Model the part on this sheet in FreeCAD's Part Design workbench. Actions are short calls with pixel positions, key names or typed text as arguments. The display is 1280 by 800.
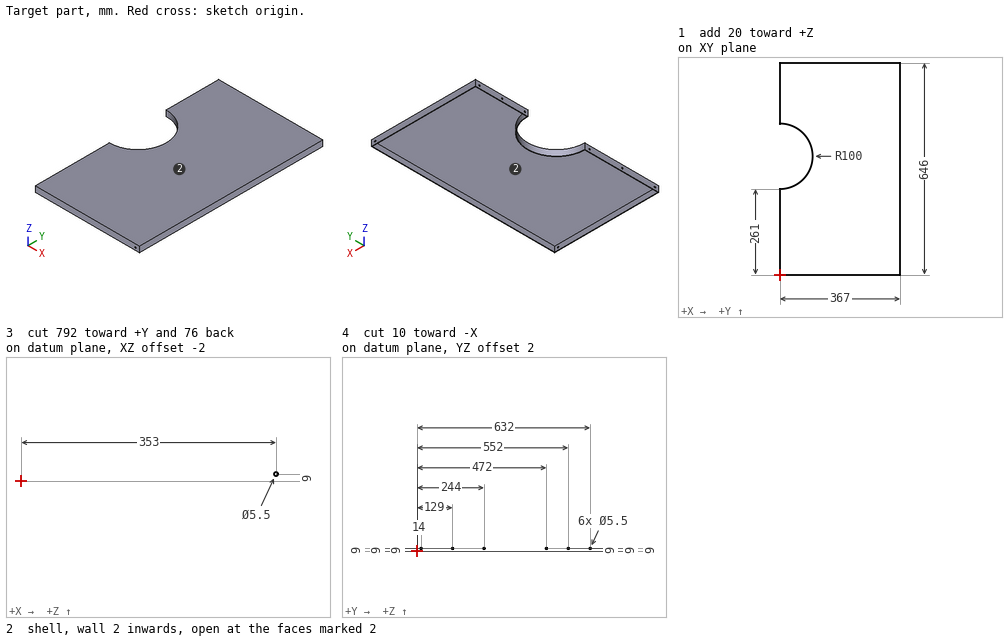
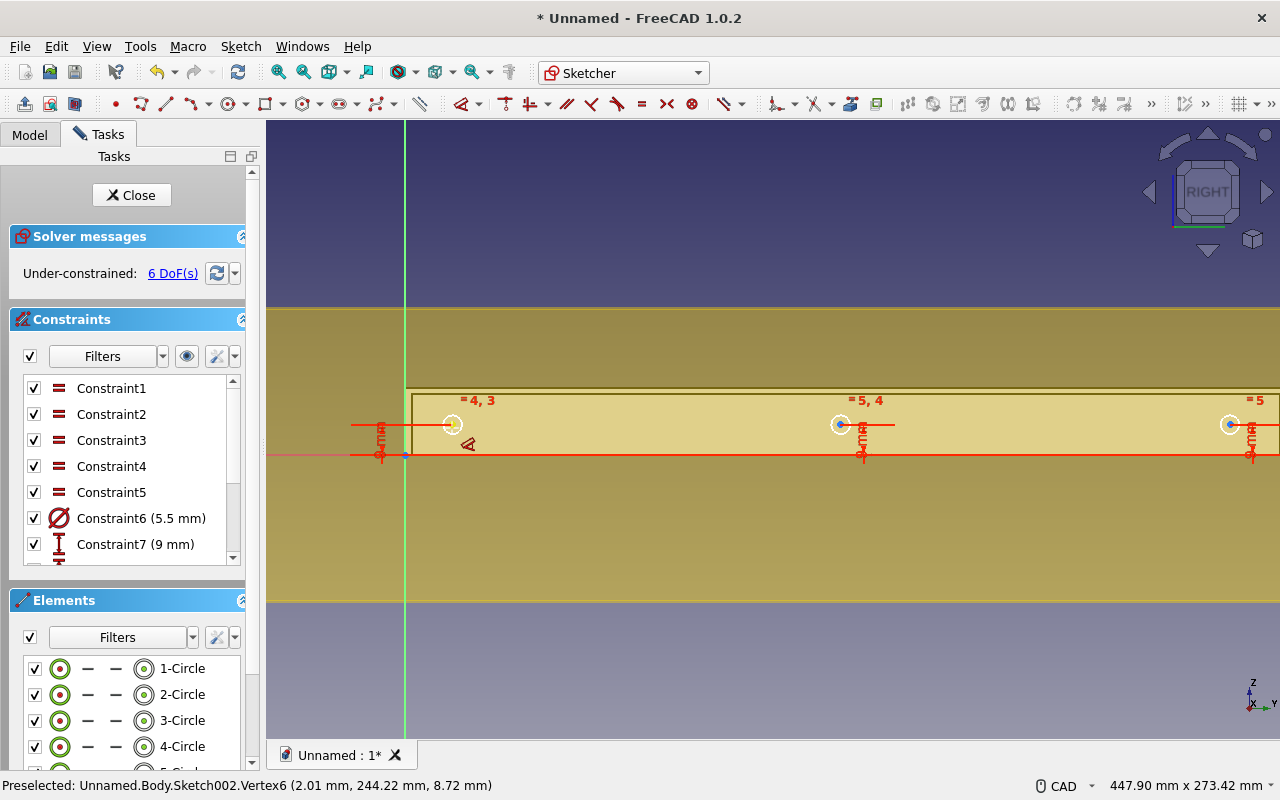
click(453, 425)
click(429, 489)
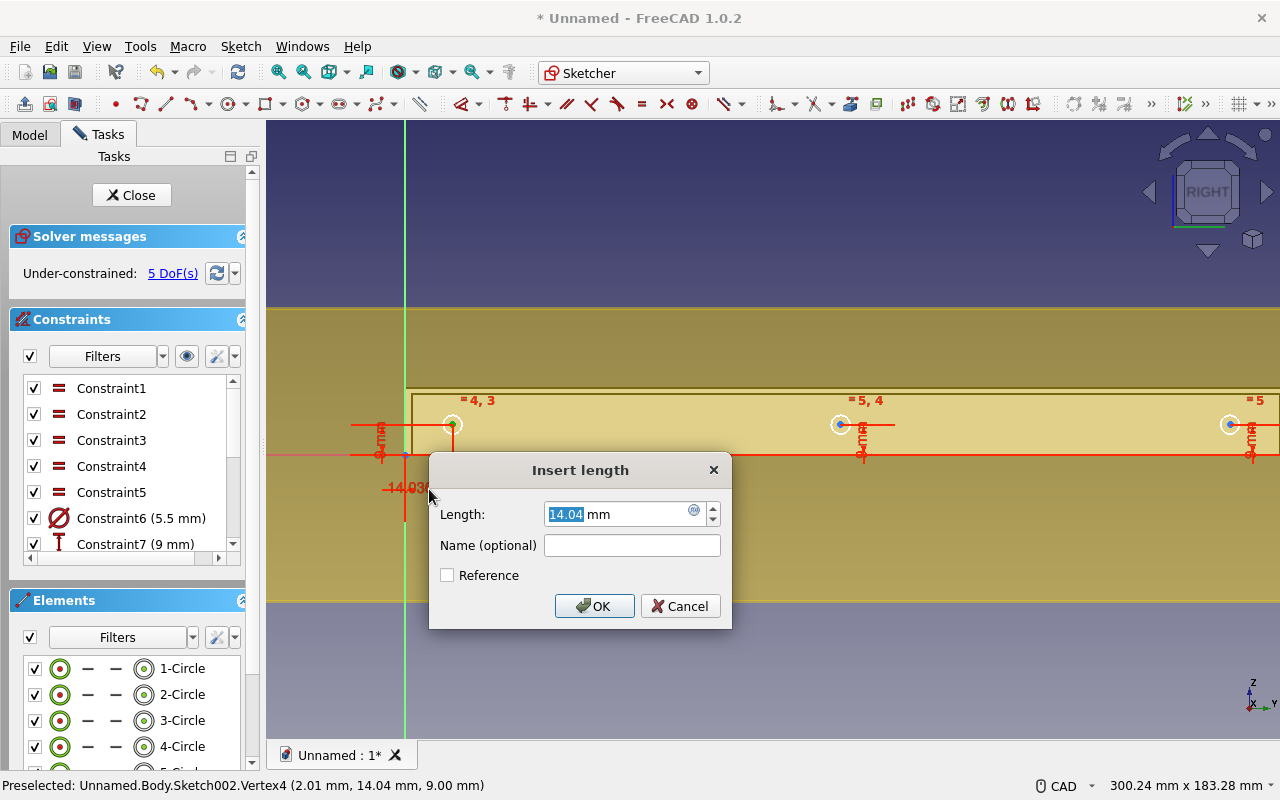
text(14)
key(Return)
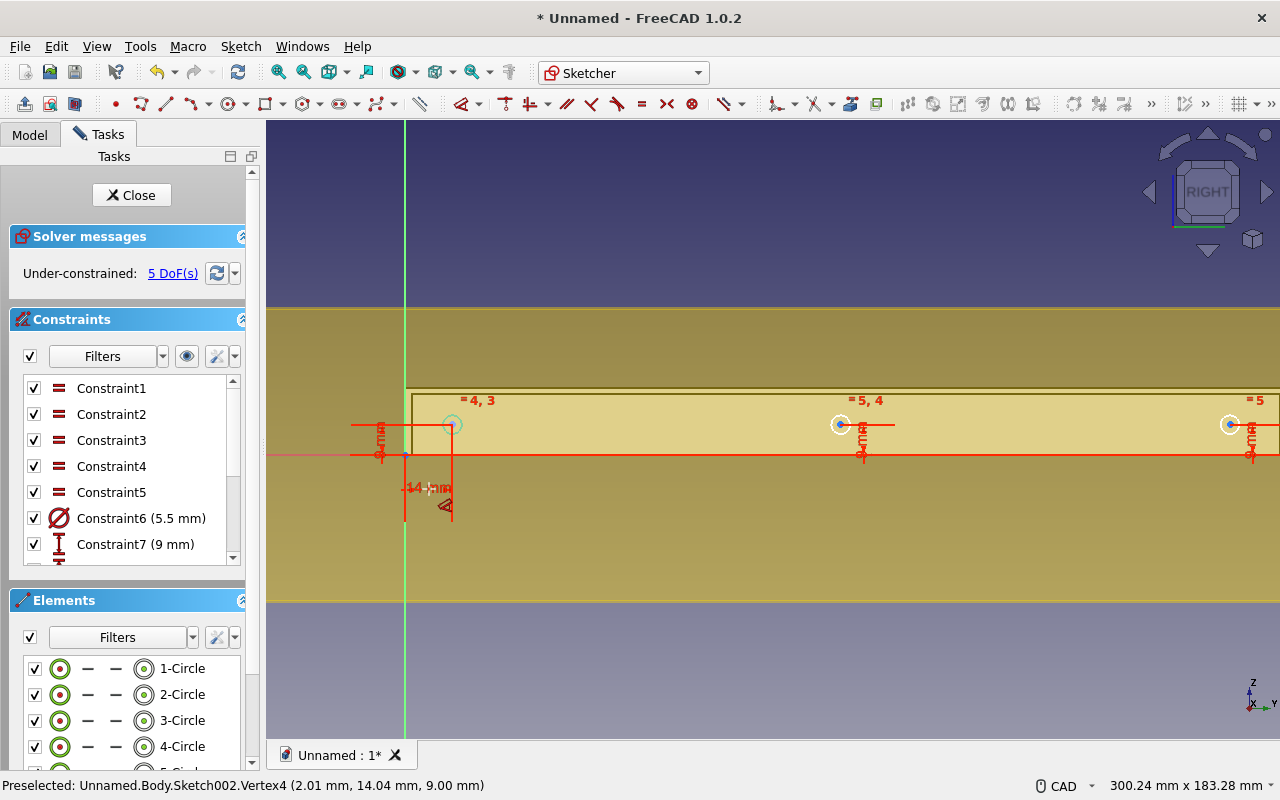
scroll(452, 428, down, 7)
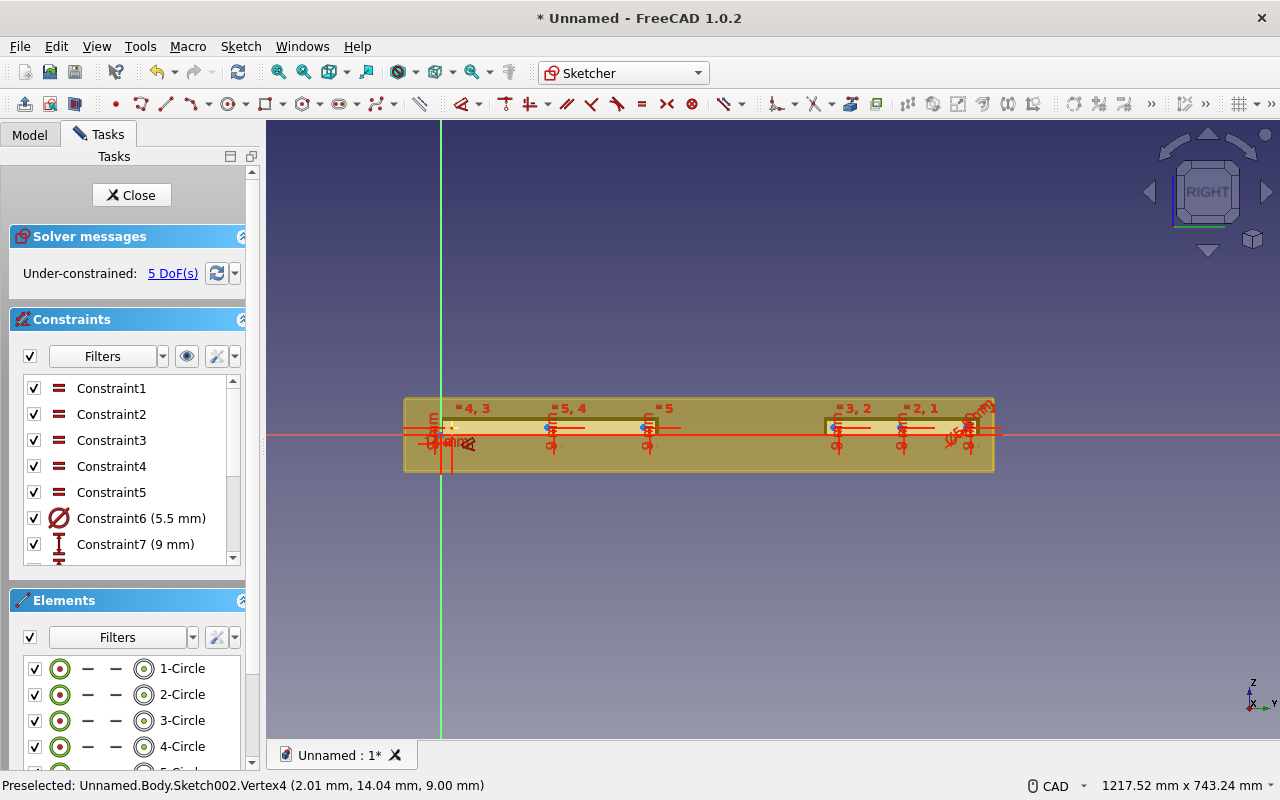
click(967, 428)
click(704, 469)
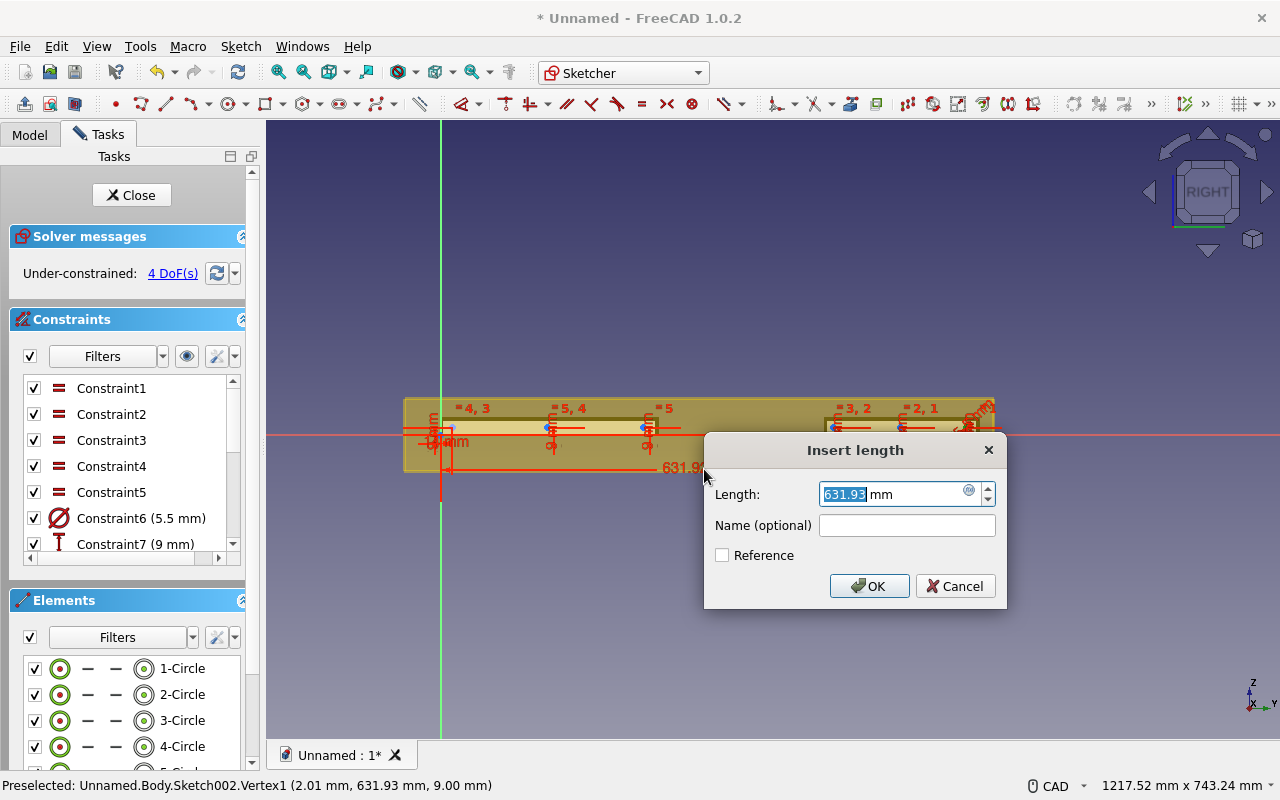
text(632)
key(Return)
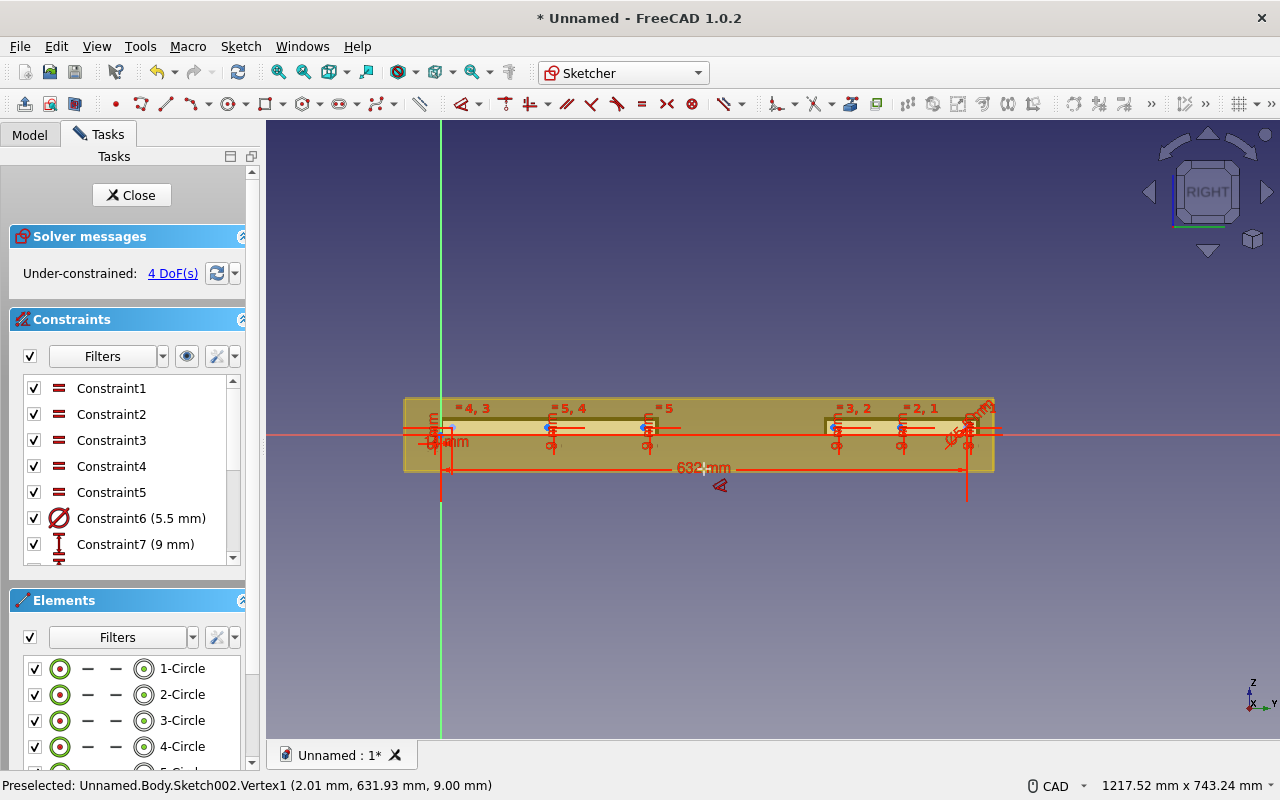
click(900, 428)
click(565, 469)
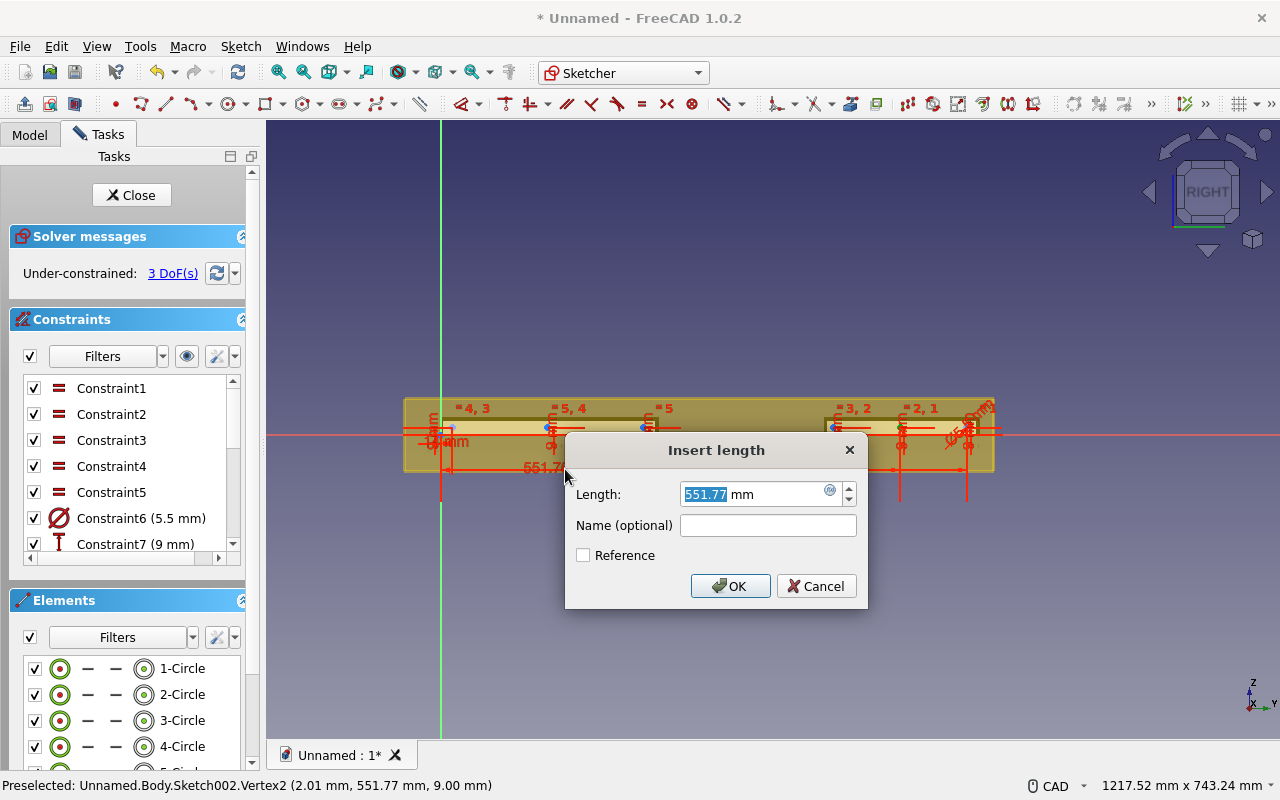
text(552)
key(Return)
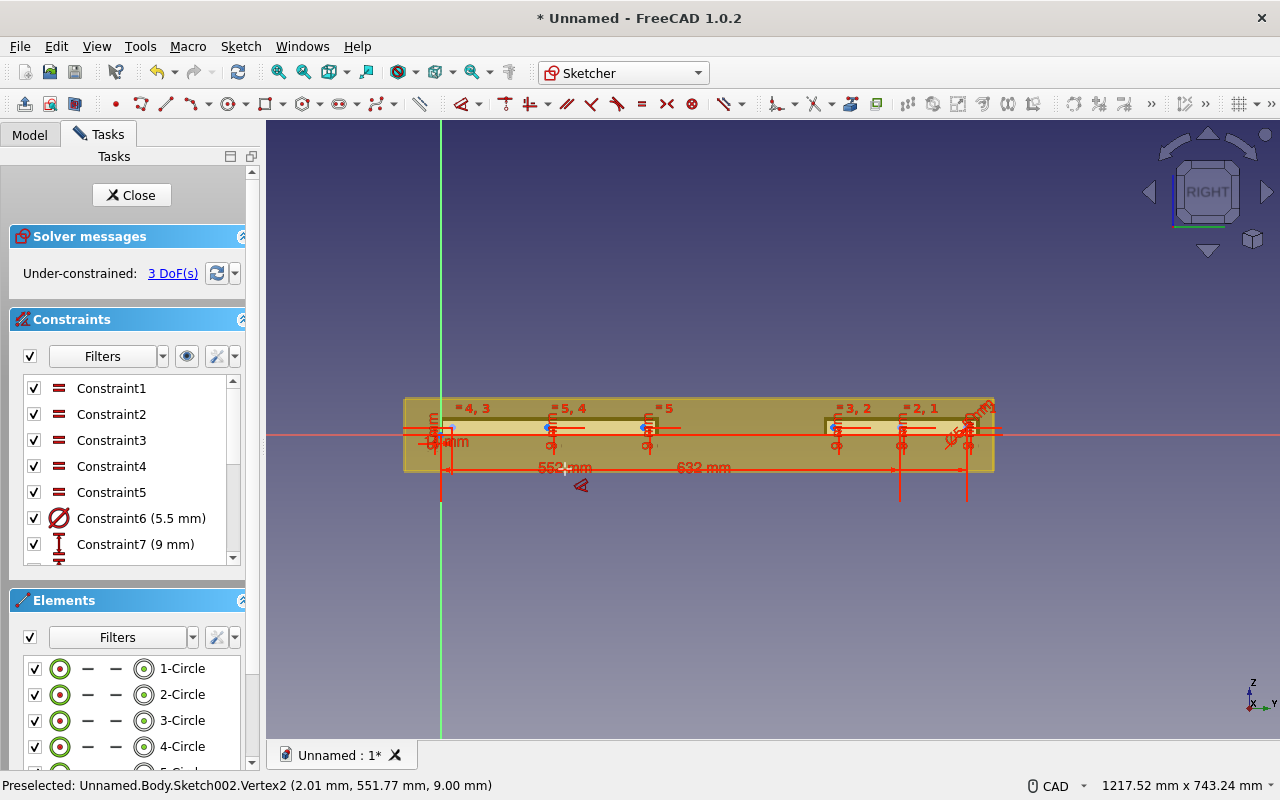
click(834, 428)
click(775, 469)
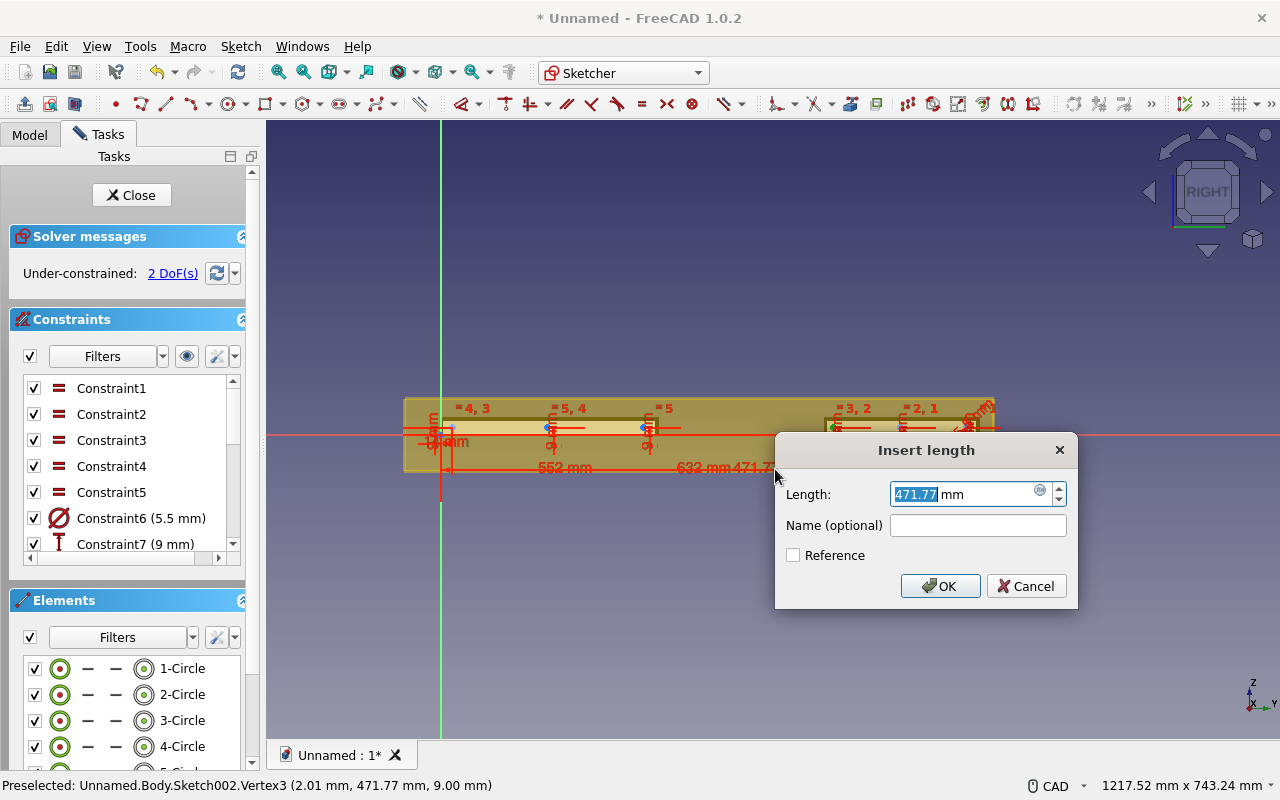
text(472)
key(Return)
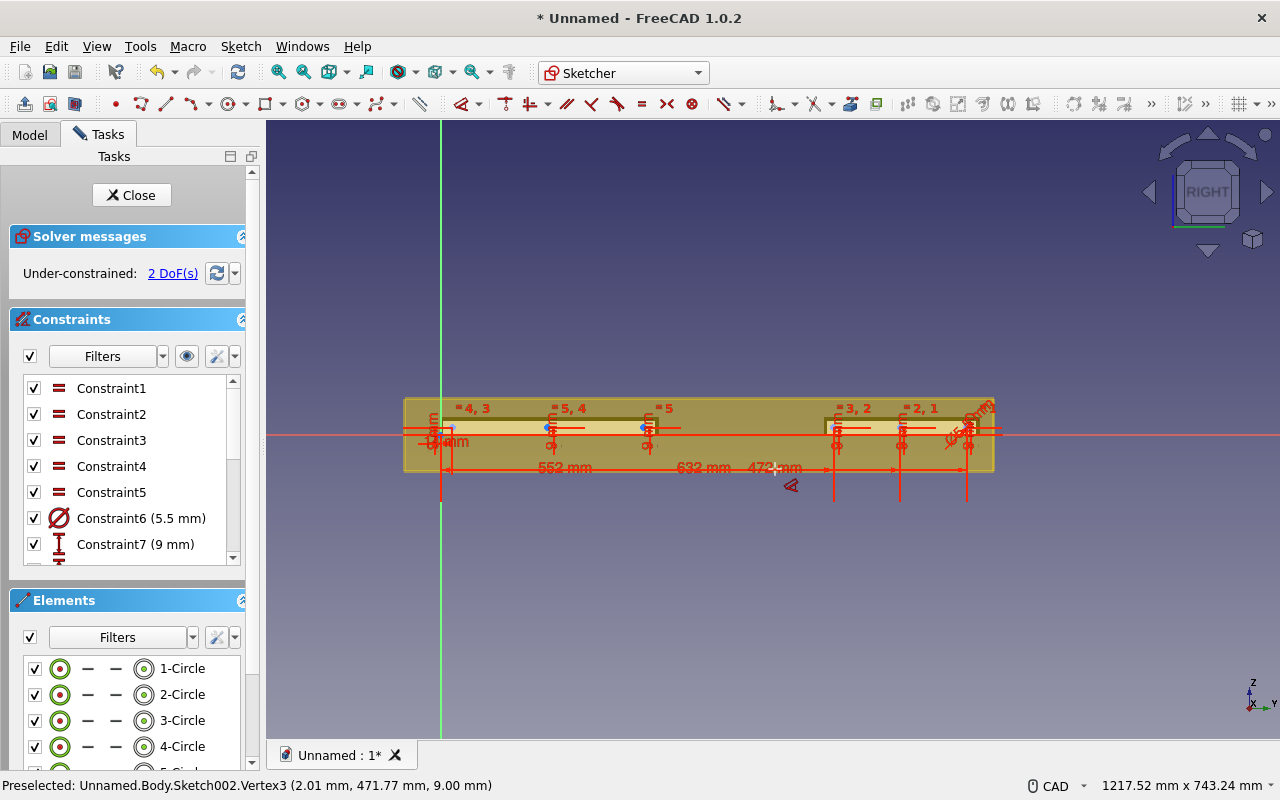
click(548, 428)
click(494, 469)